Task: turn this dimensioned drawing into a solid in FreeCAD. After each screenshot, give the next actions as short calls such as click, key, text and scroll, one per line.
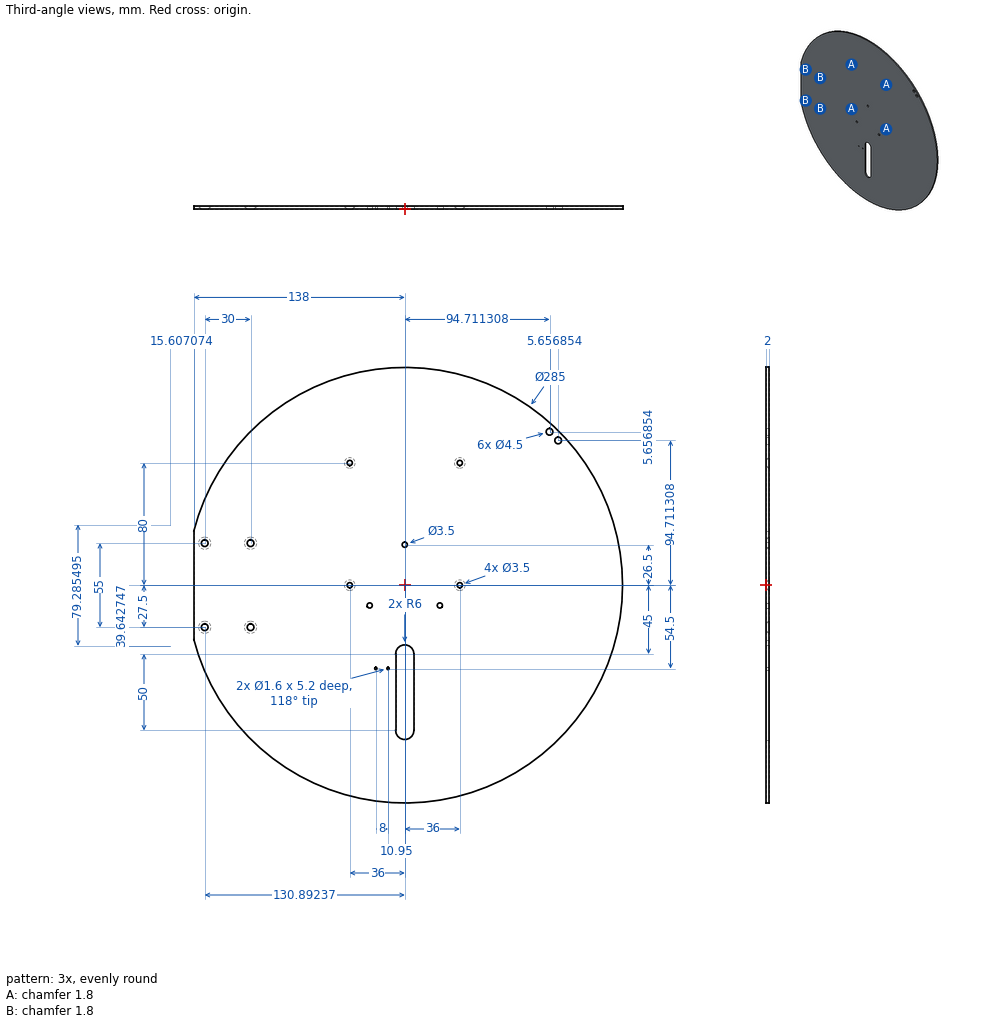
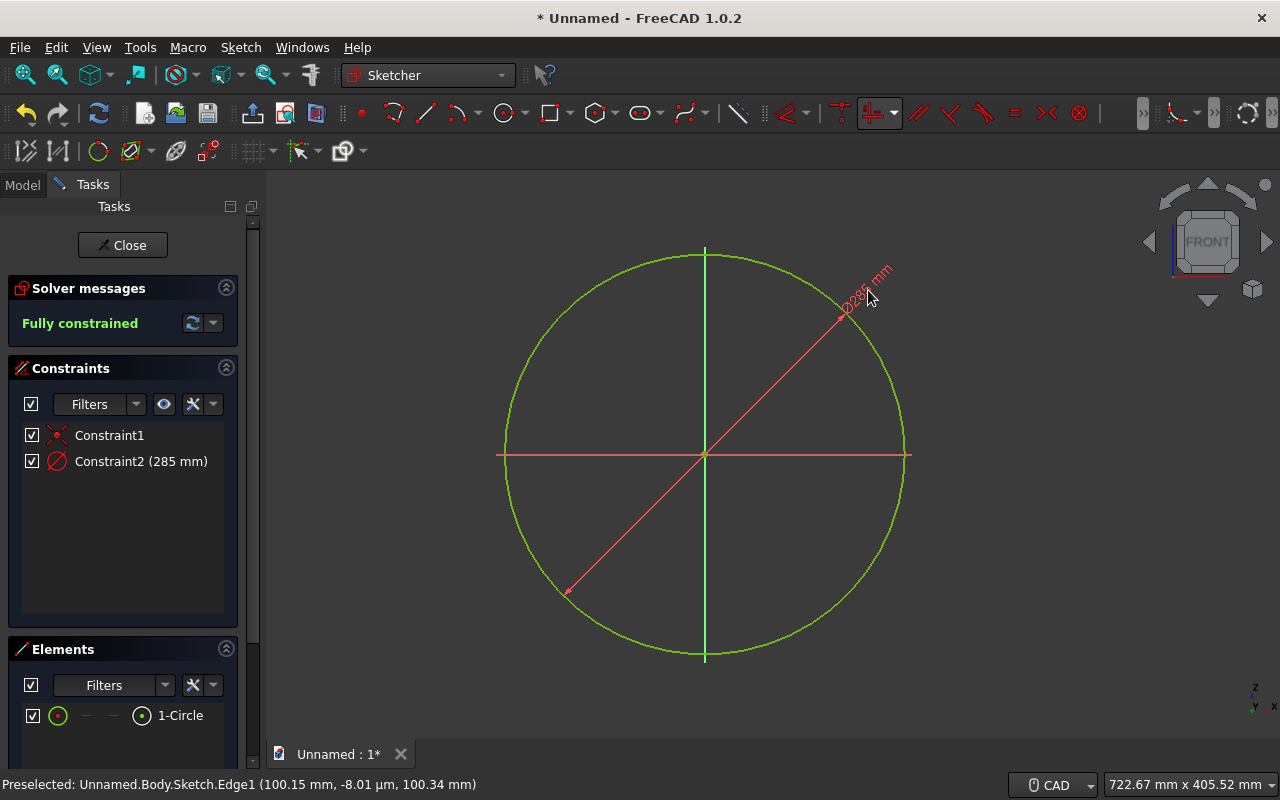
click(123, 245)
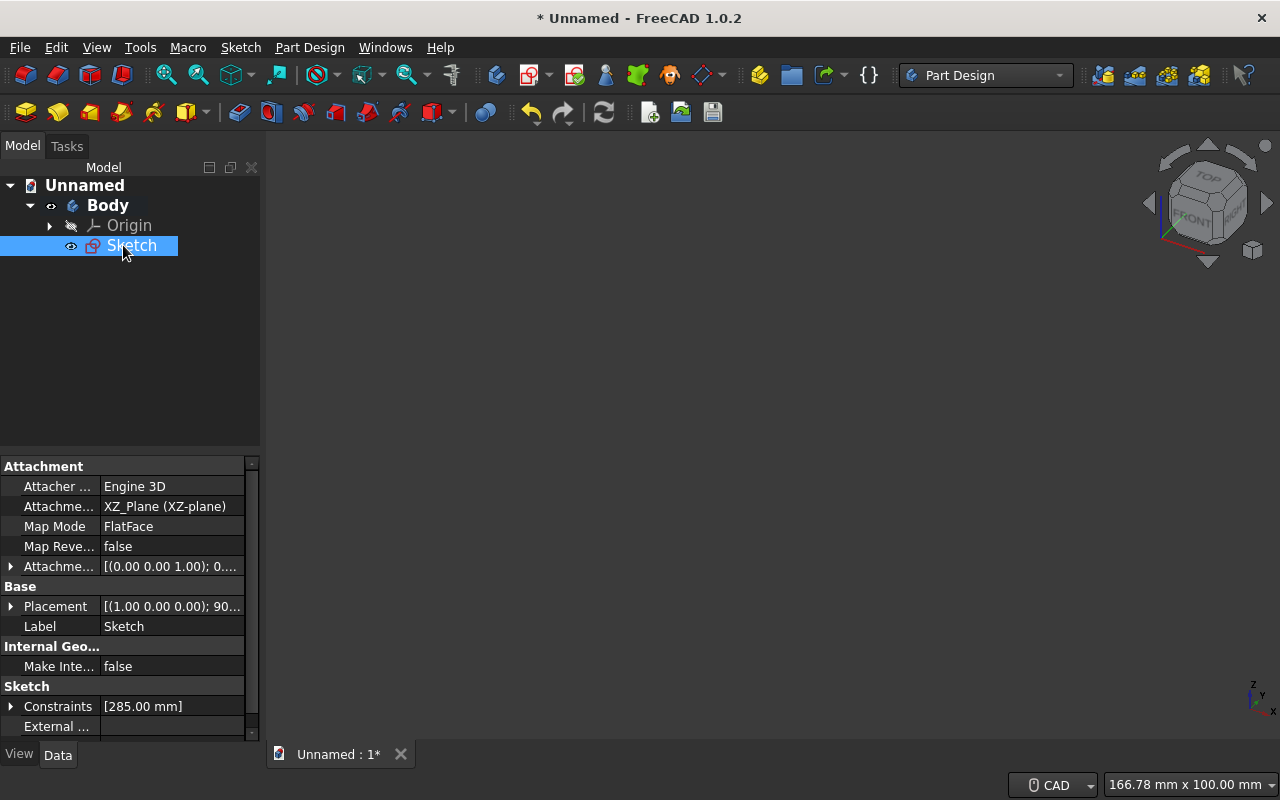
click(26, 112)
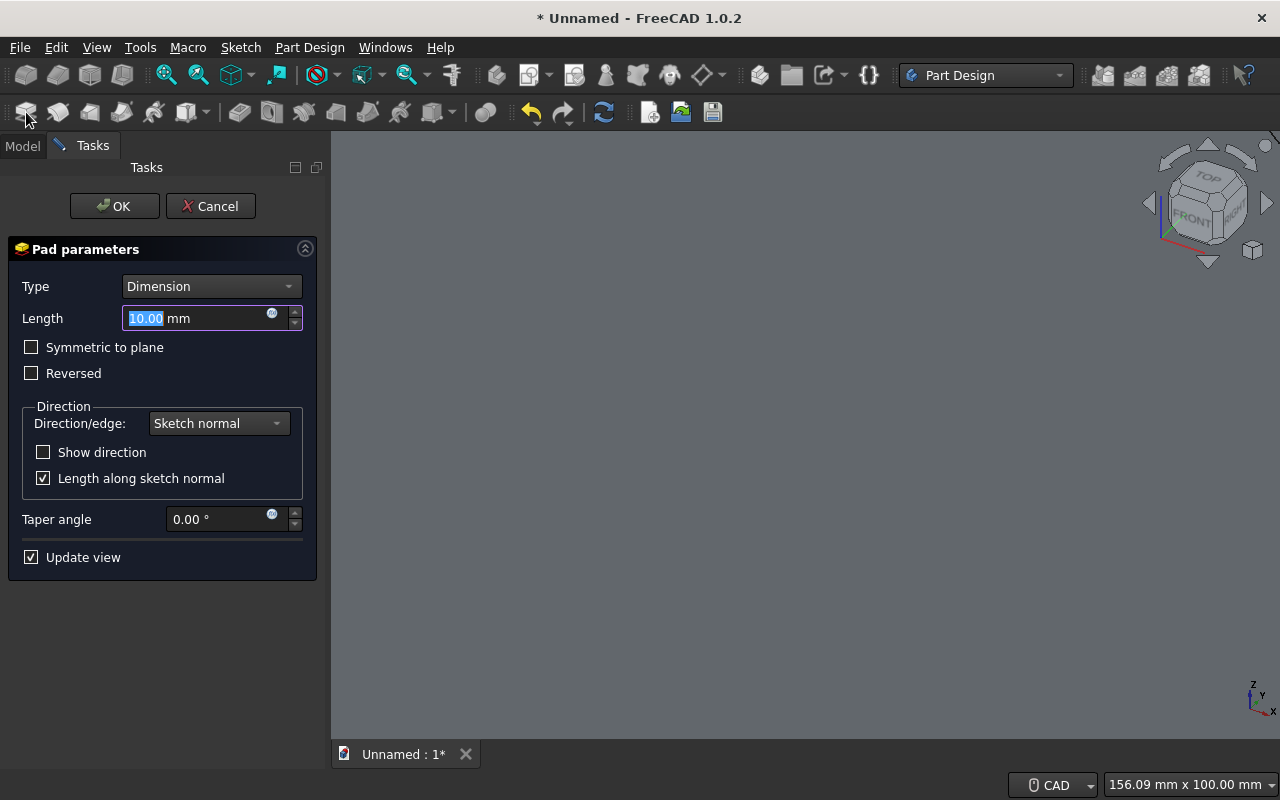
text(2)
key(Tab)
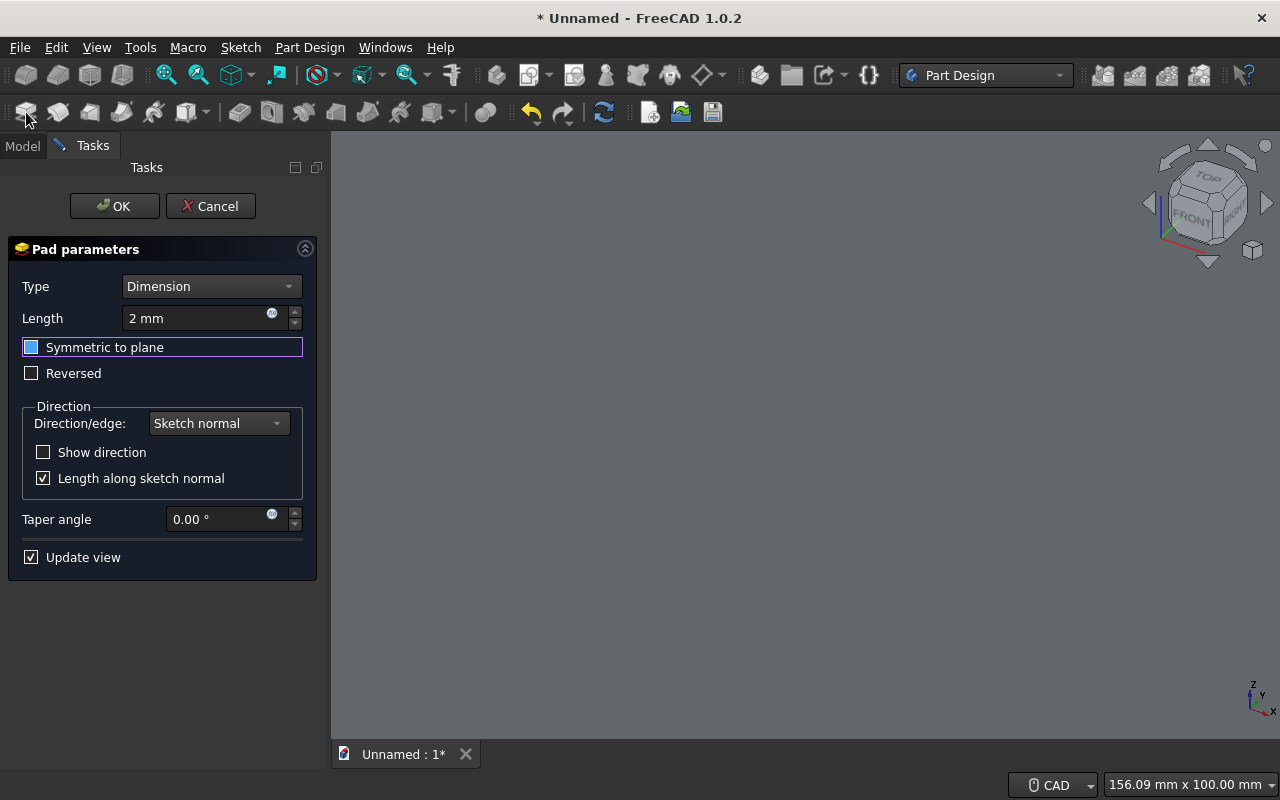
click(30, 373)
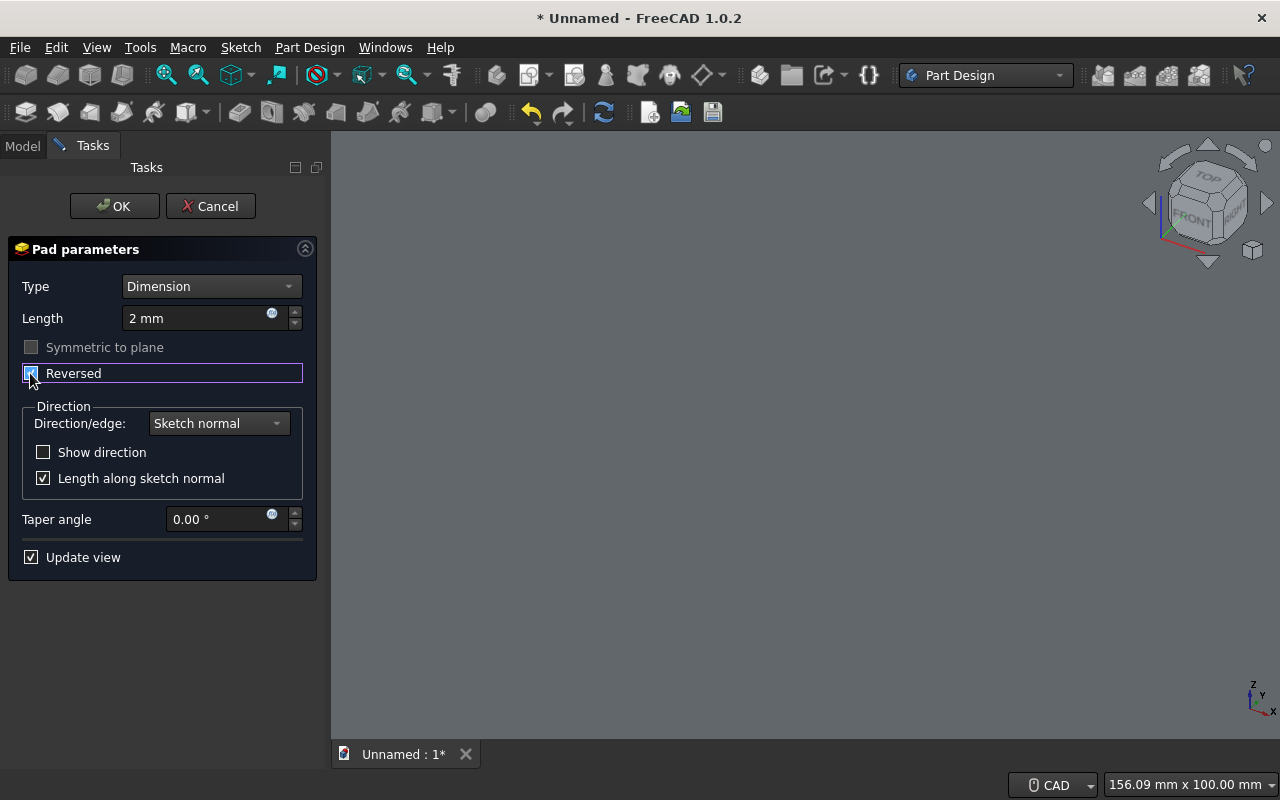
click(115, 206)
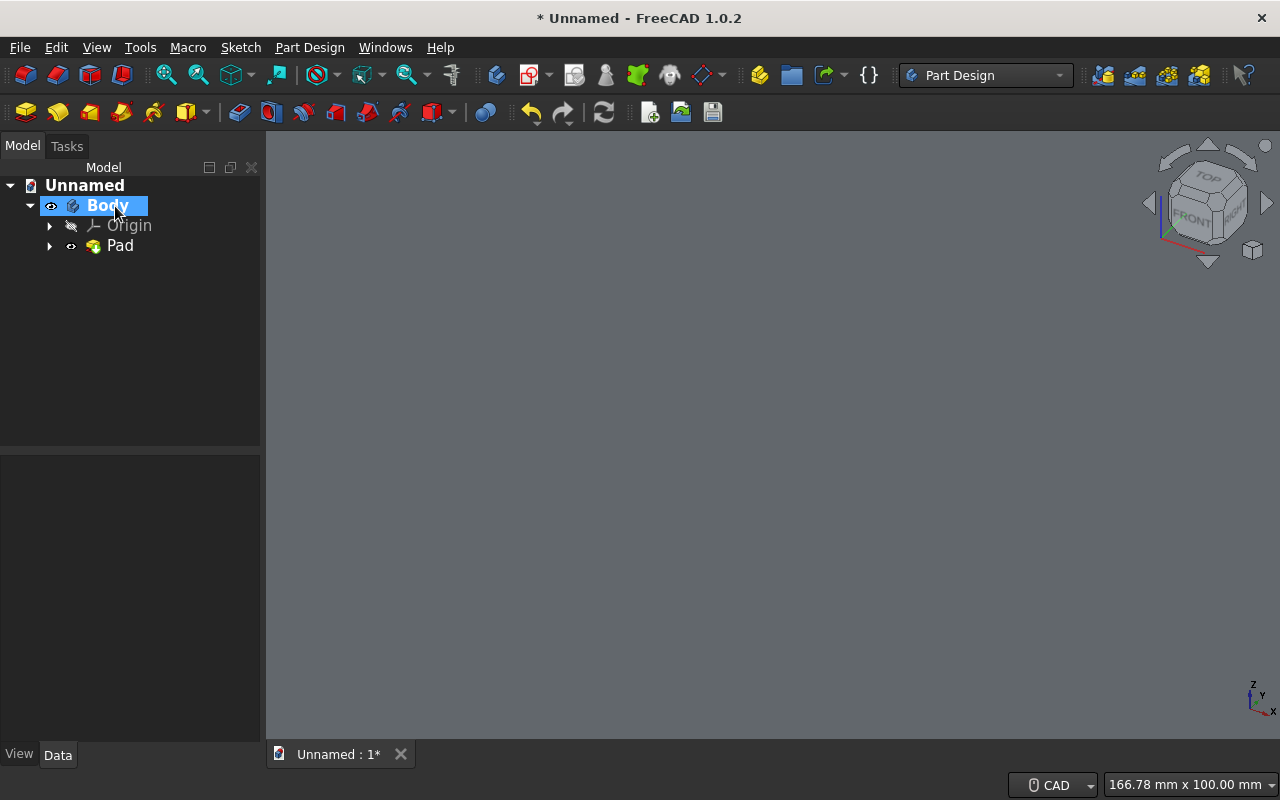
key(v)
key(f)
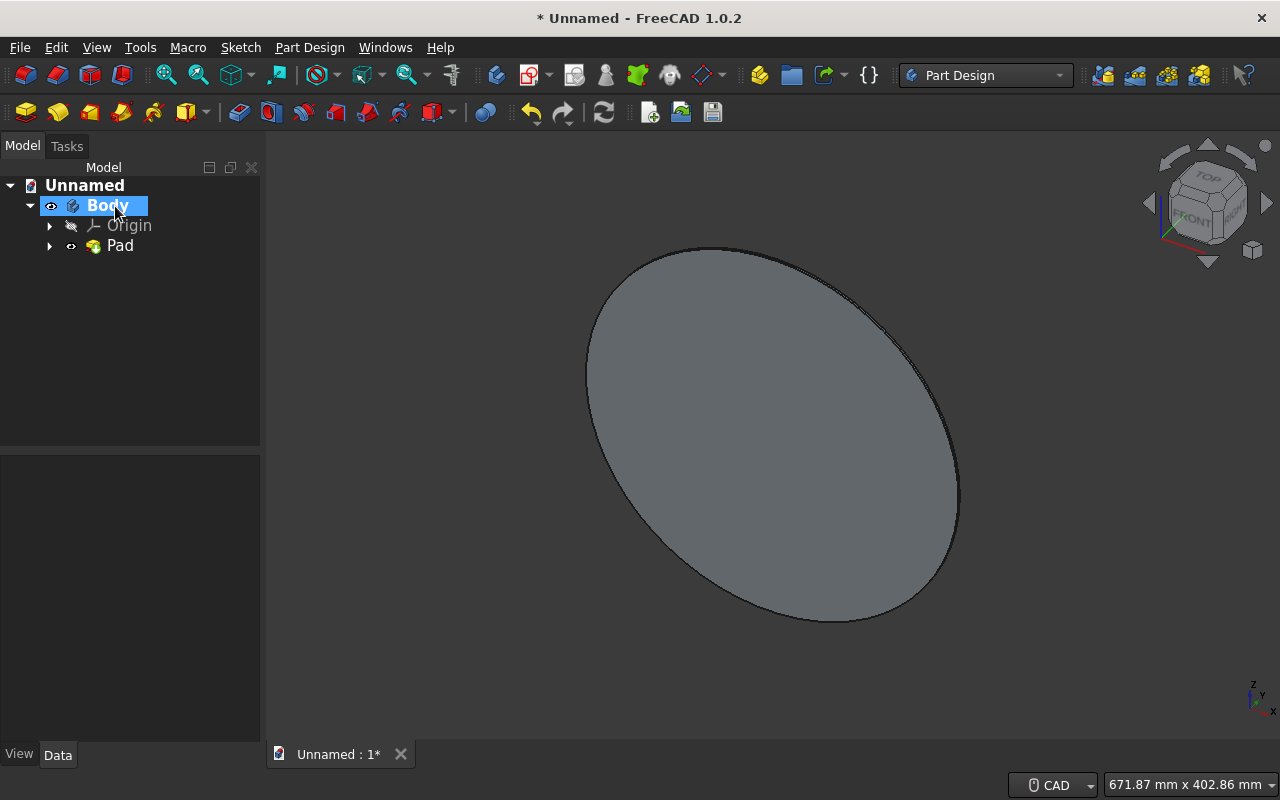
key(4)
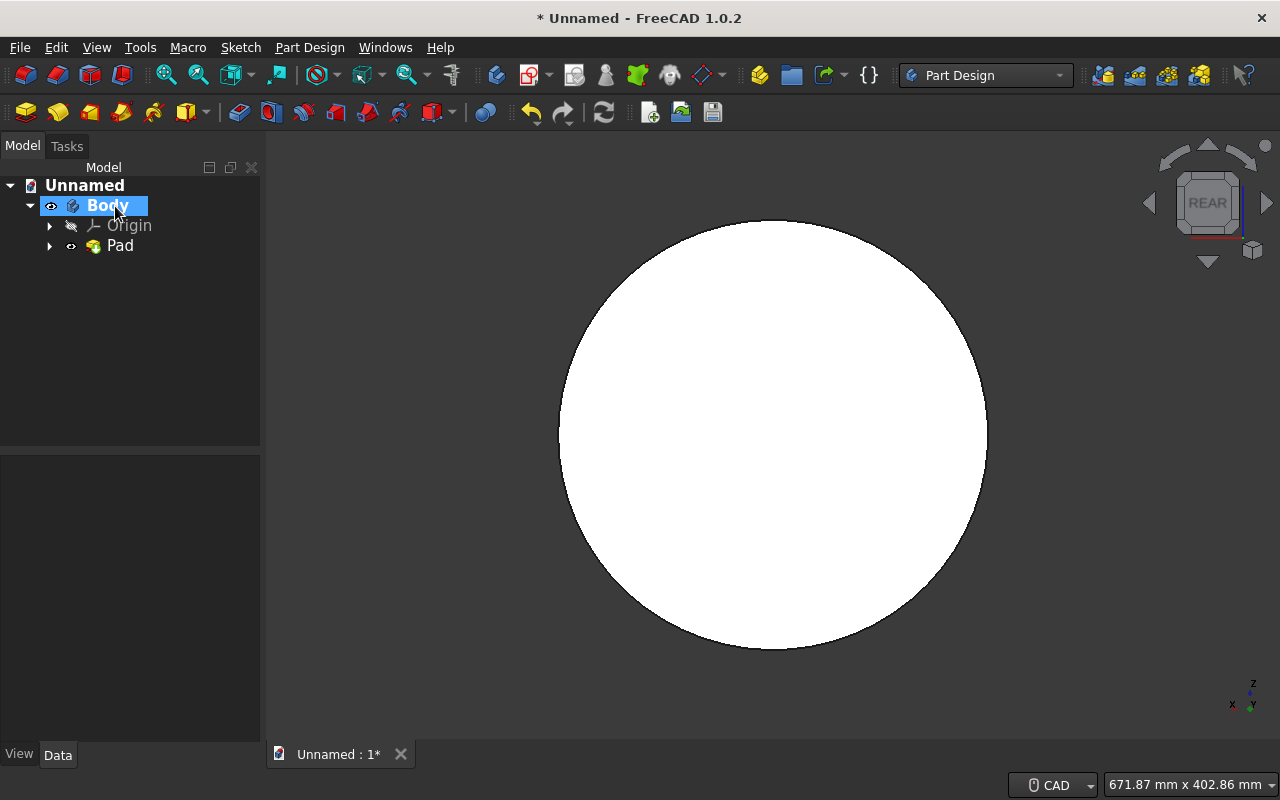
click(773, 434)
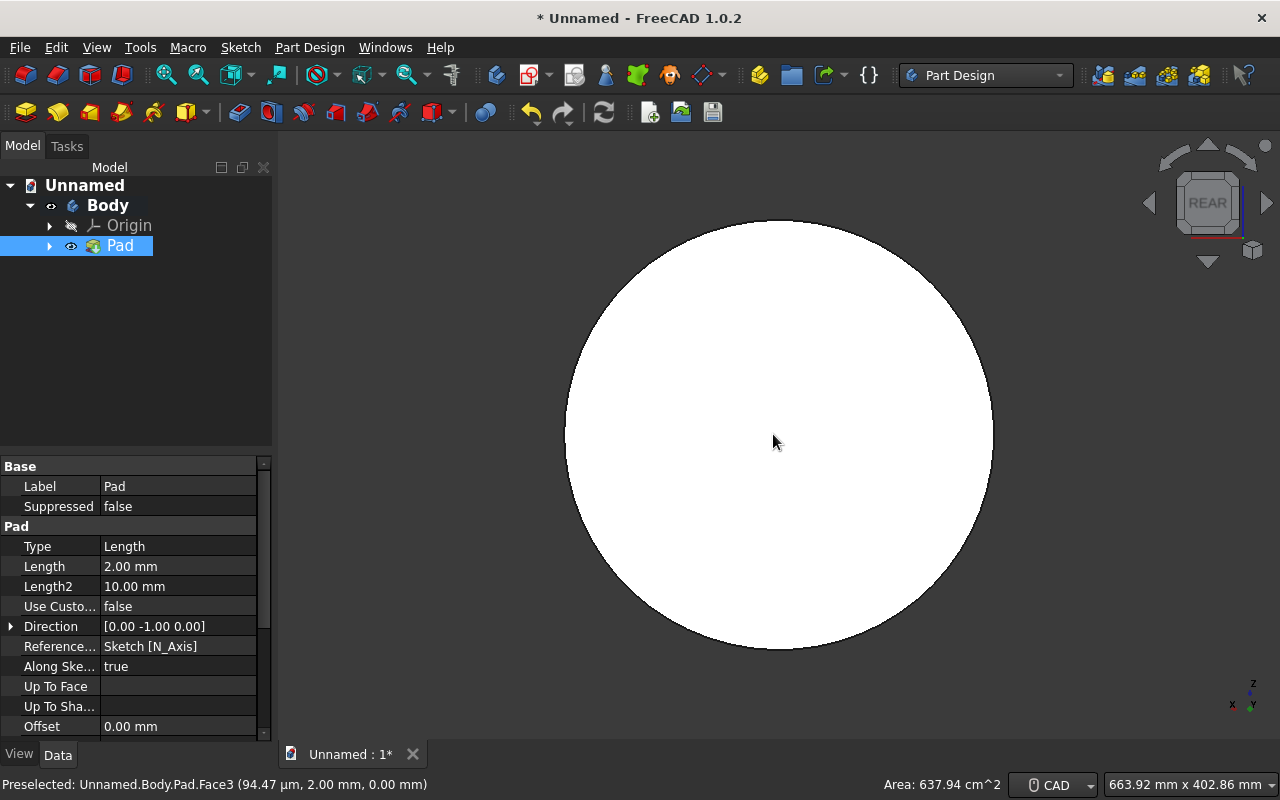
click(530, 76)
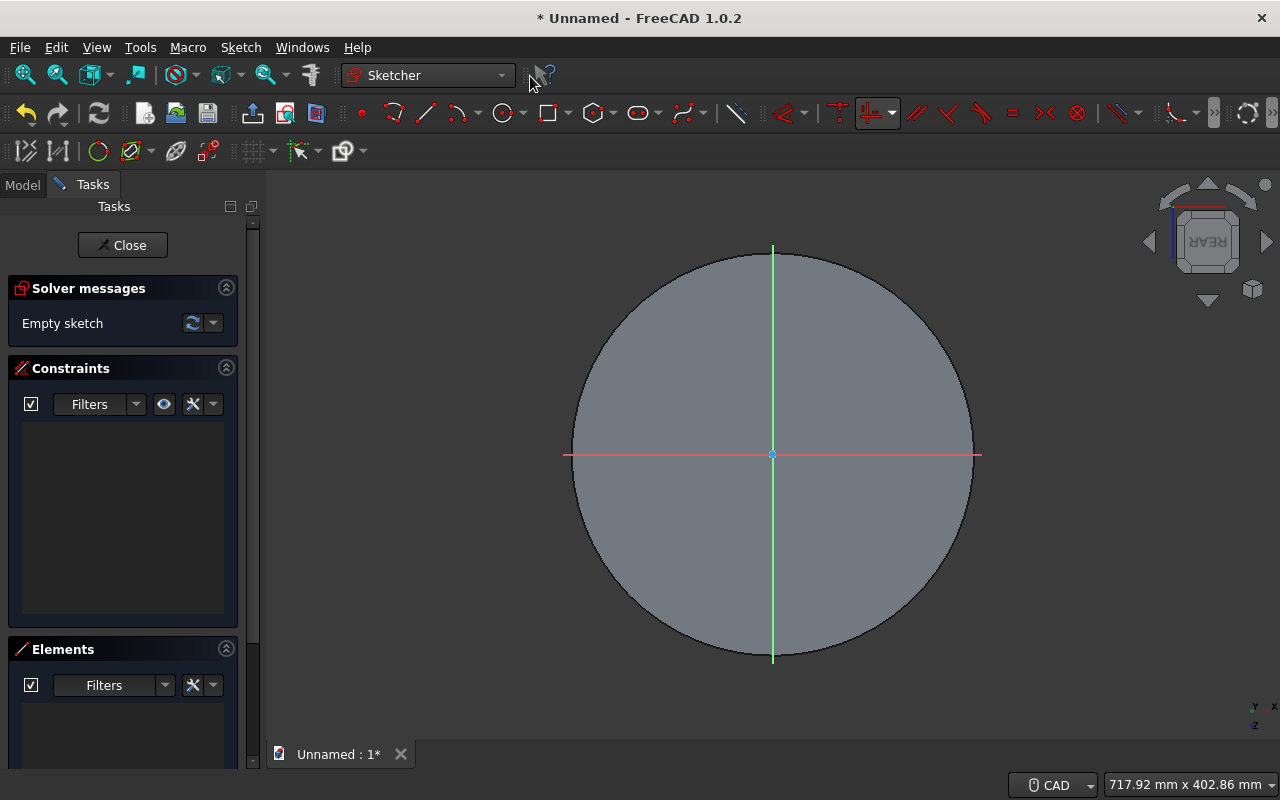
scroll(776, 494, up, 15)